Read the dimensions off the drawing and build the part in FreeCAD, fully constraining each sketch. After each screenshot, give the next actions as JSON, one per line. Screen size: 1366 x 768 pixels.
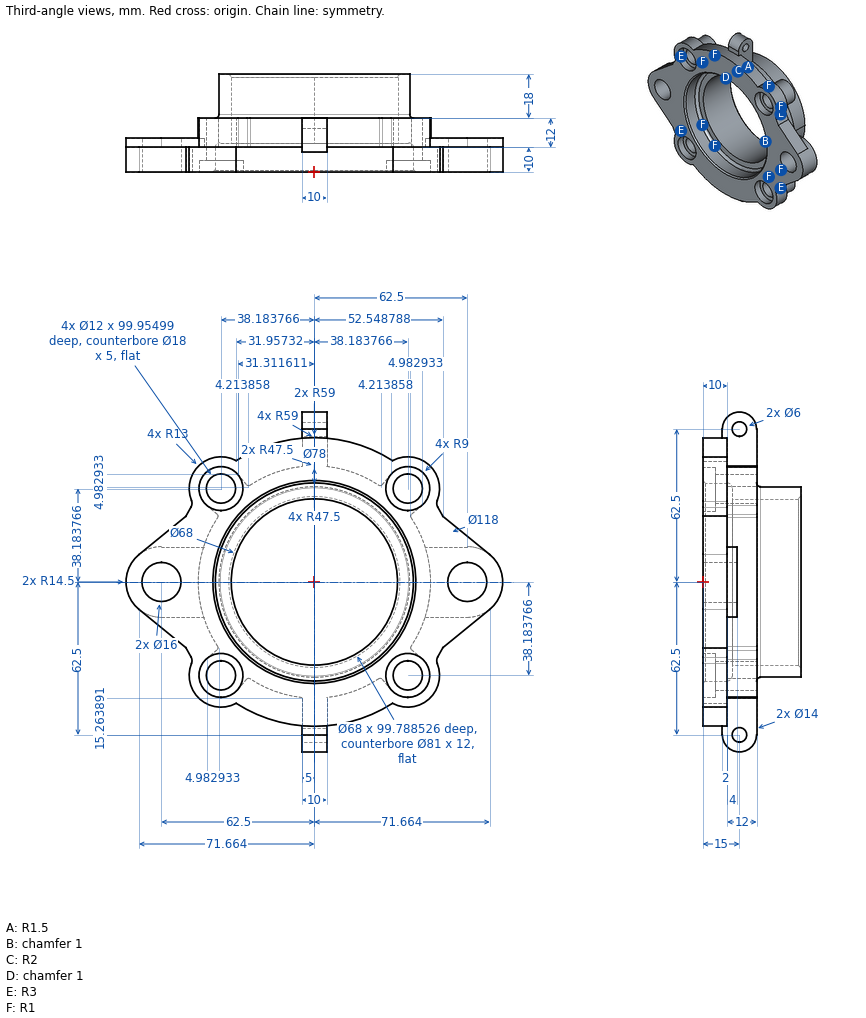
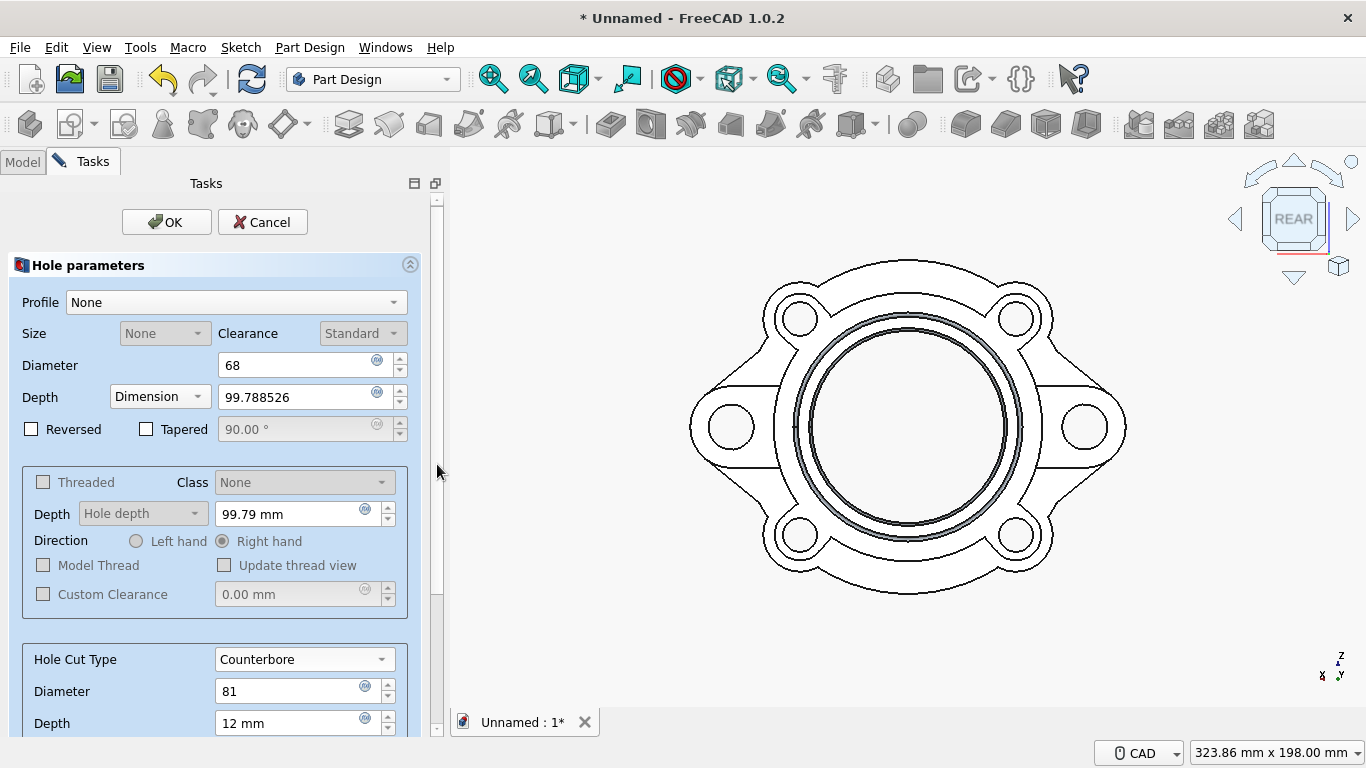
{"action": "left_click", "coordinate": [167, 222]}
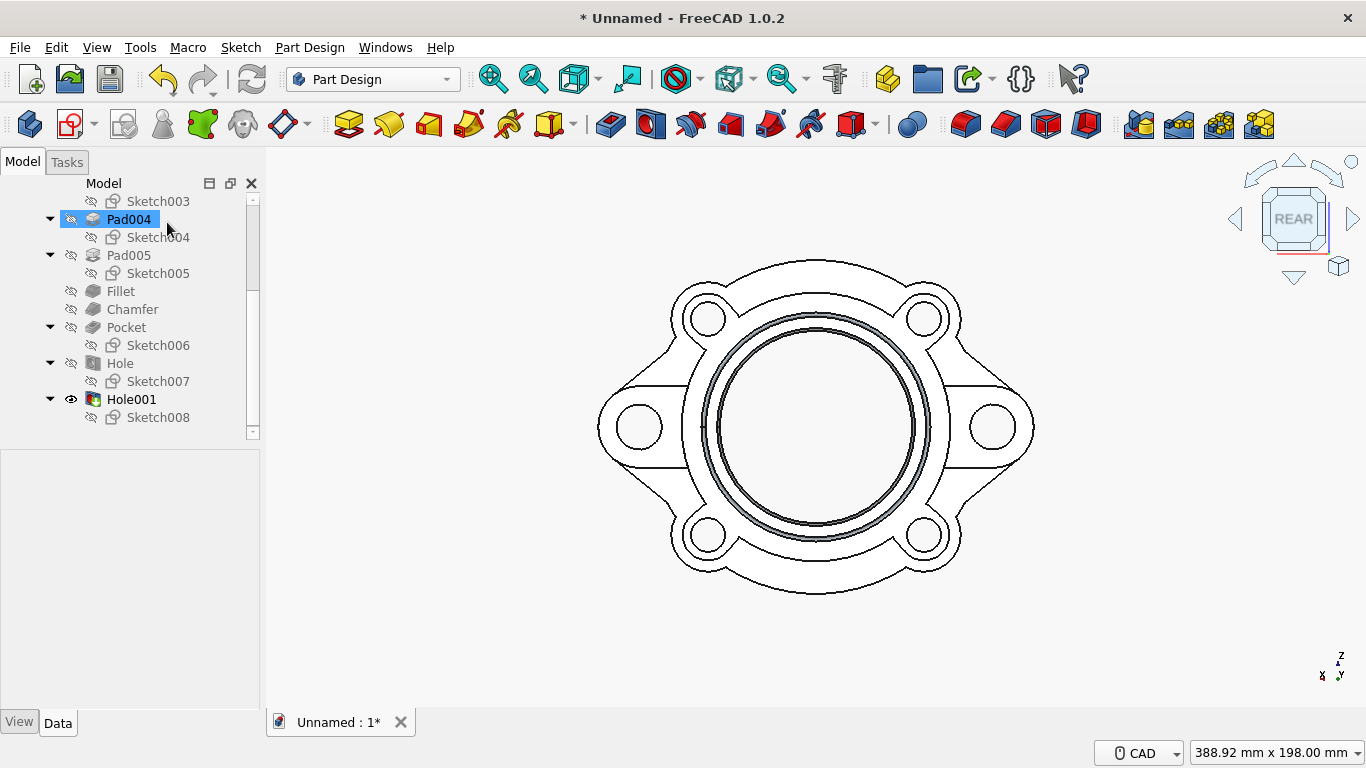
{"action": "key", "text": "0"}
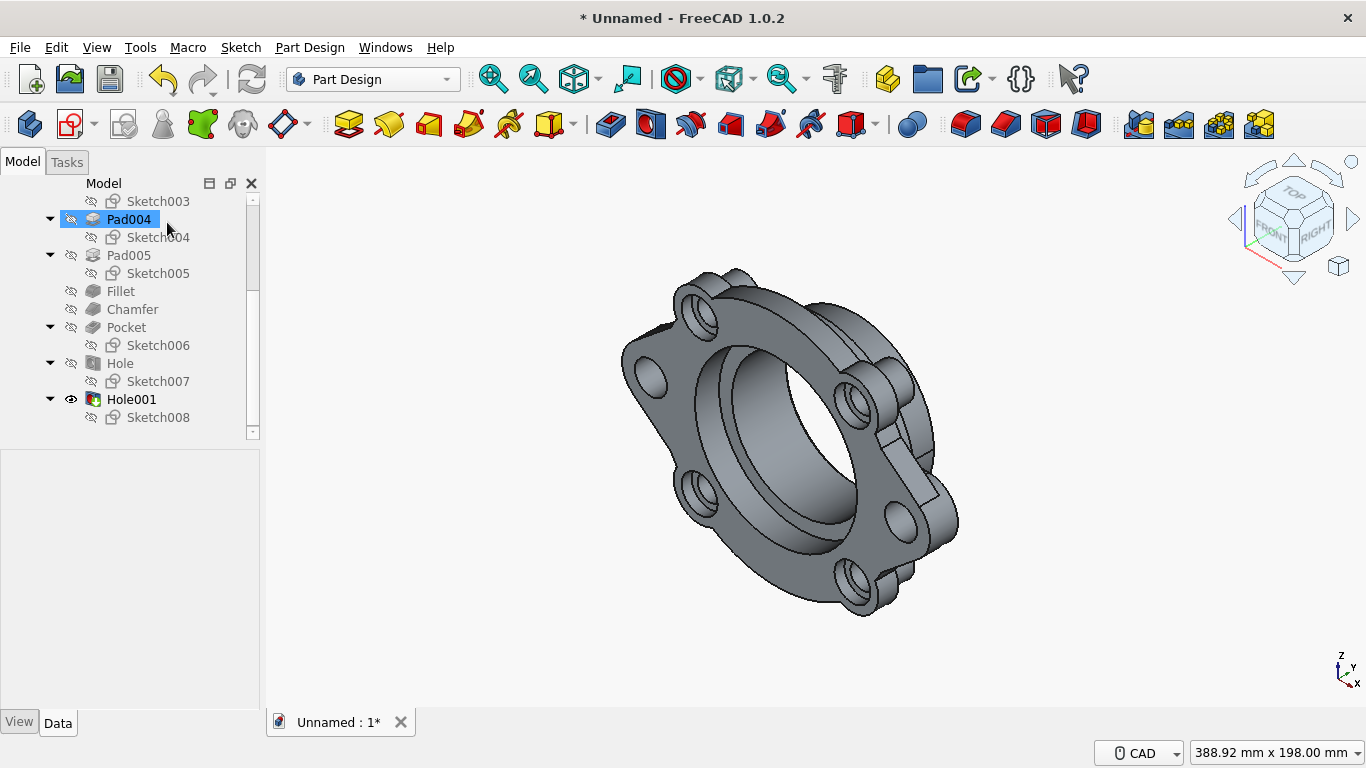
{"action": "key", "text": "2"}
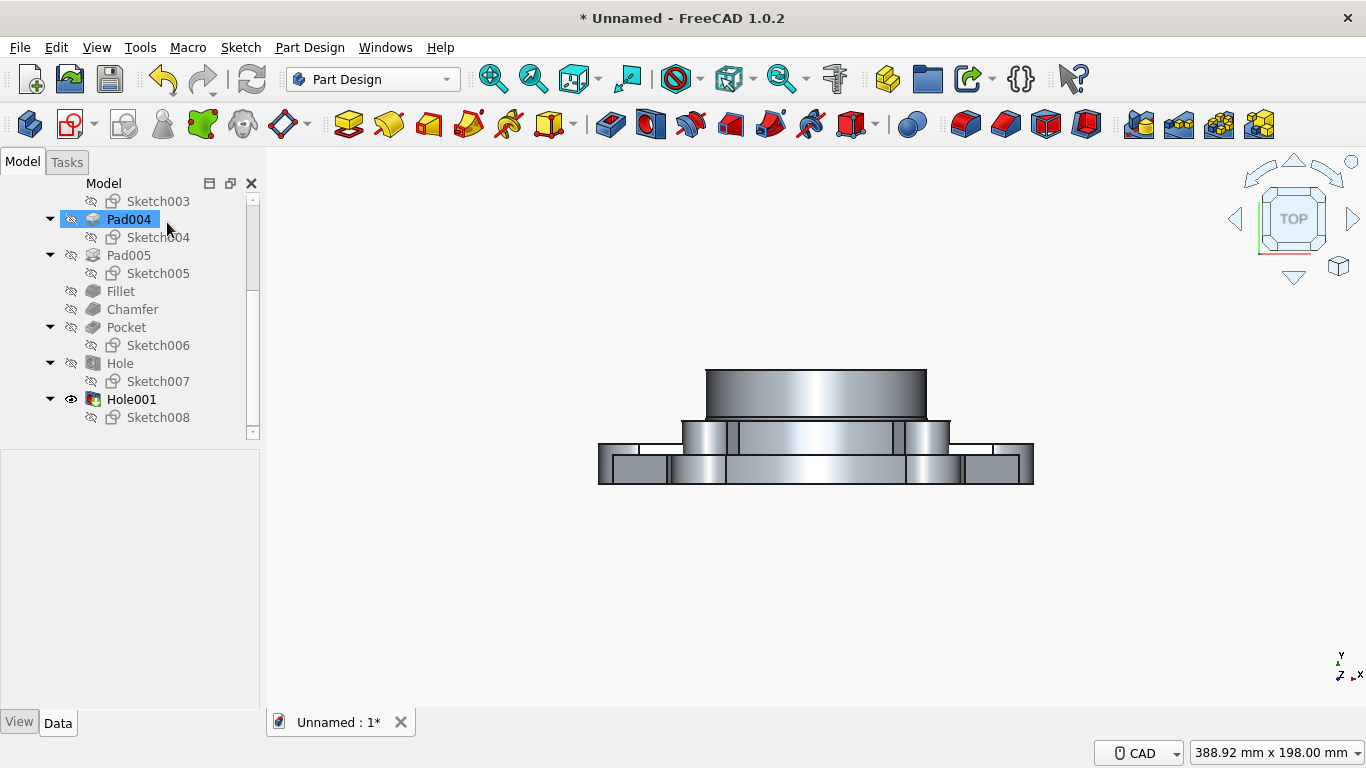
{"action": "left_click", "coordinate": [494, 80]}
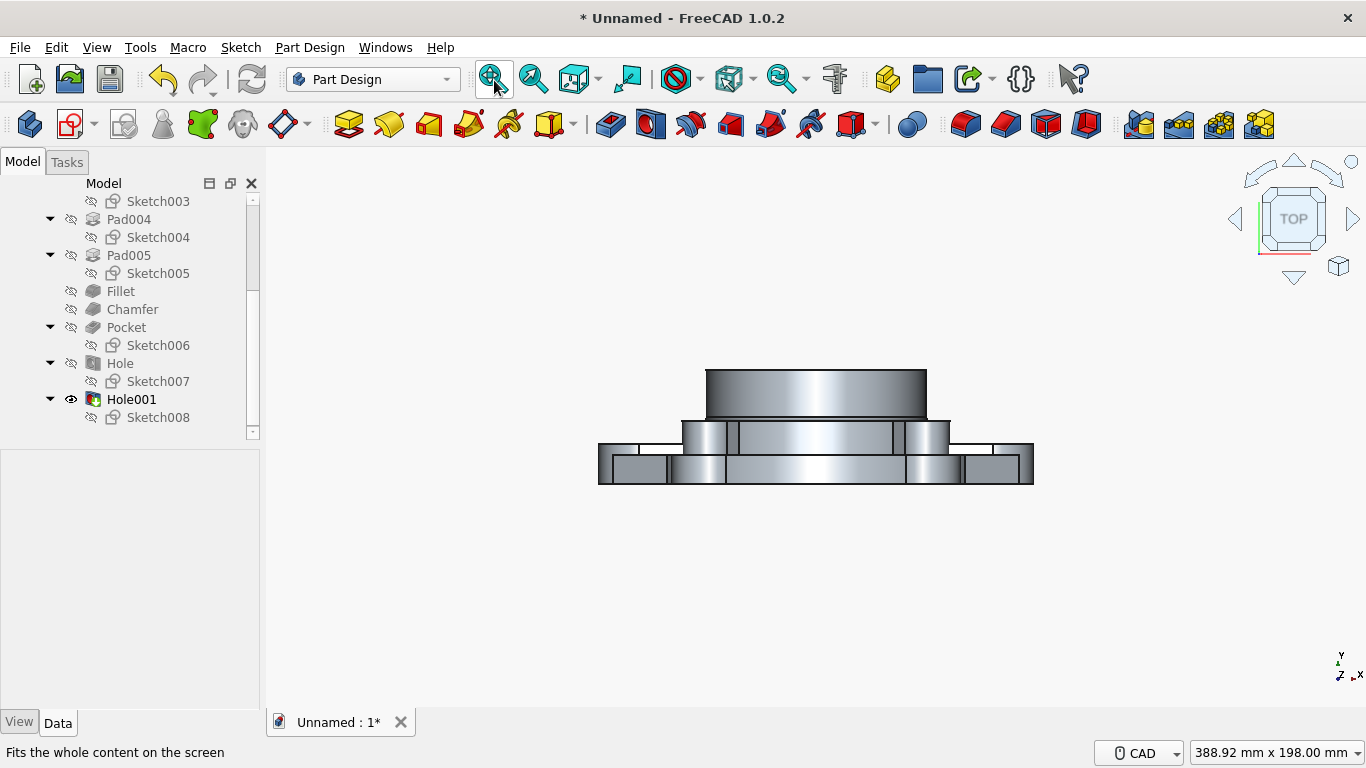
{"action": "key", "text": "1"}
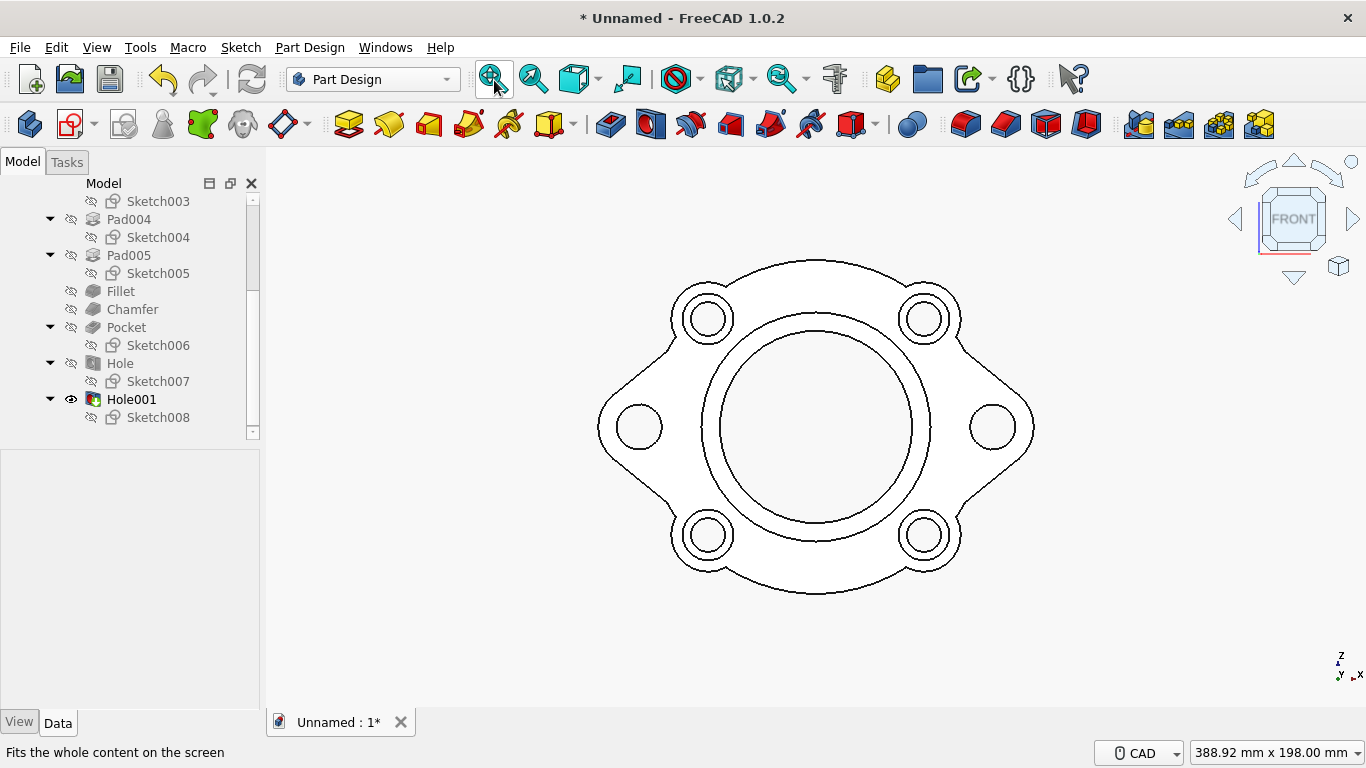
{"action": "key", "text": "3"}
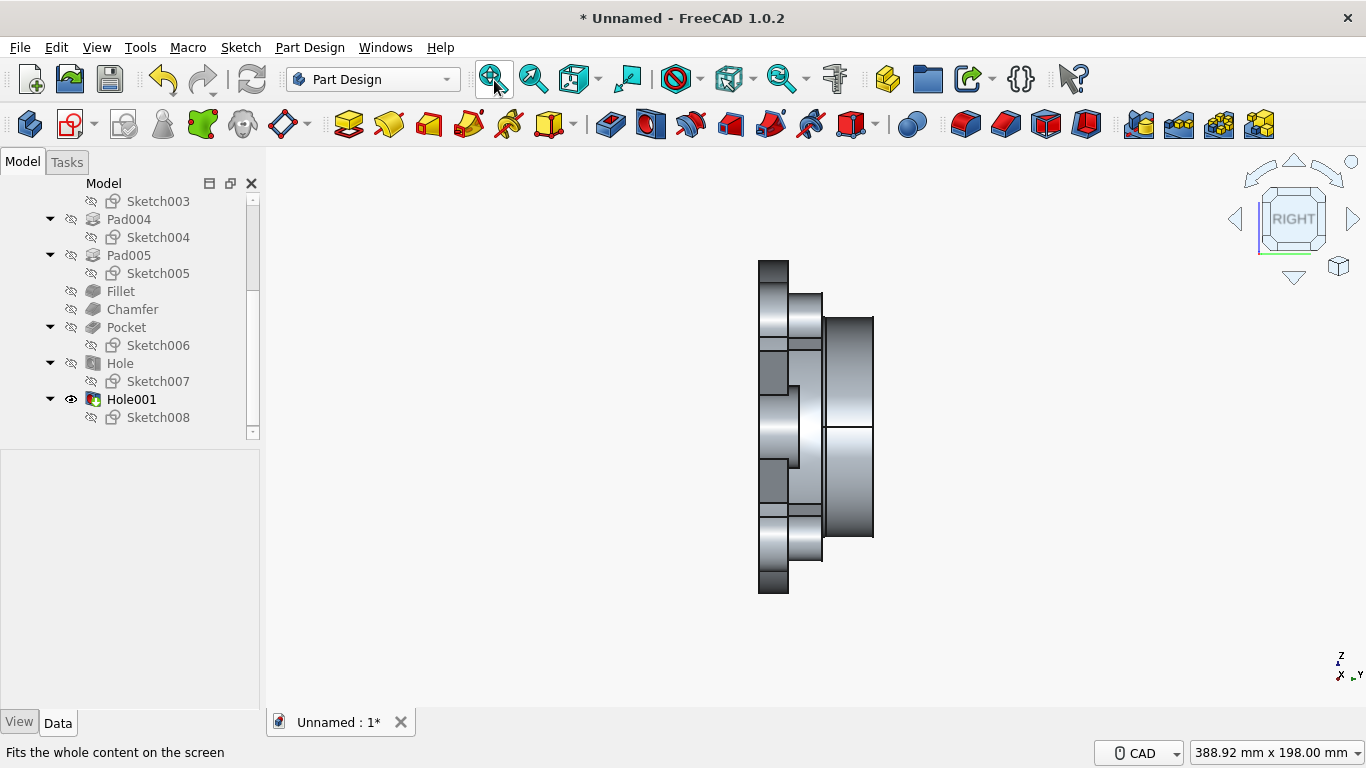
{"action": "key", "text": "5"}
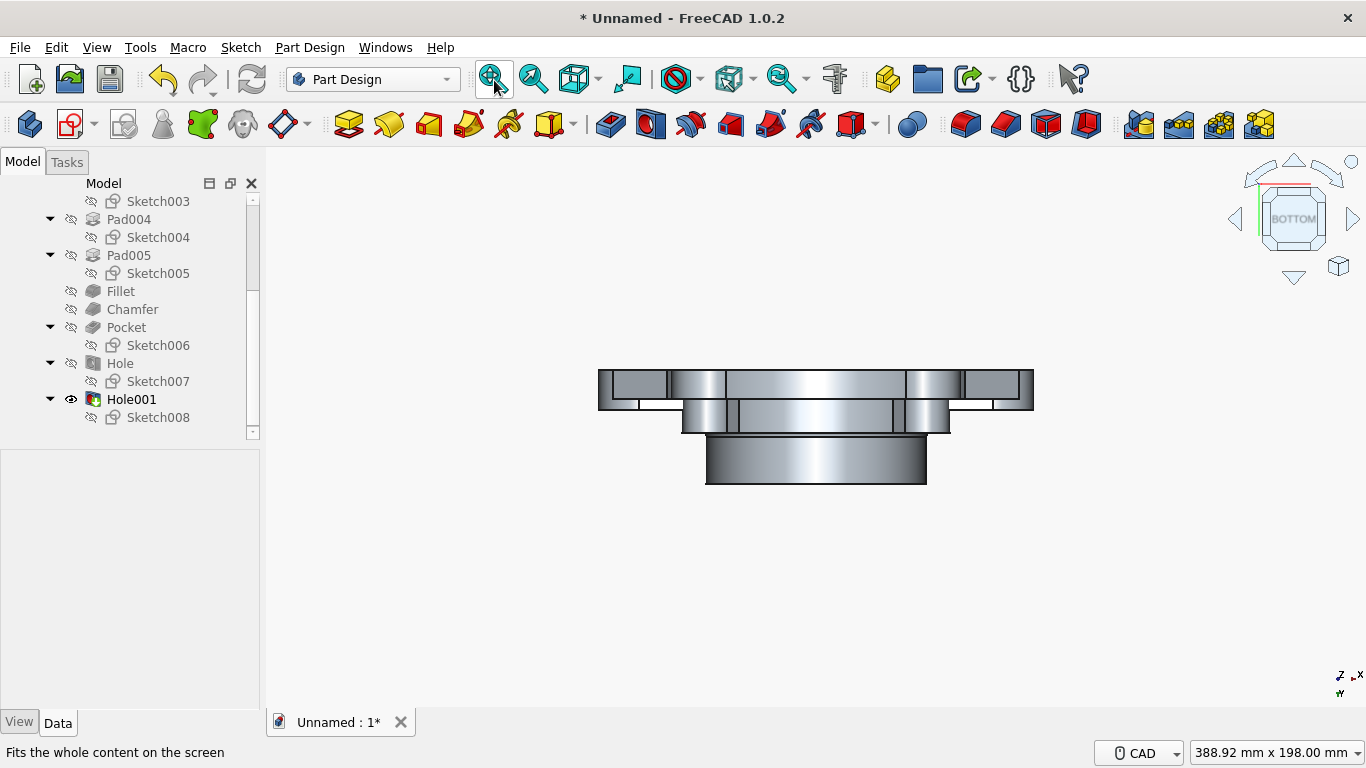
{"action": "left_click", "coordinate": [494, 80]}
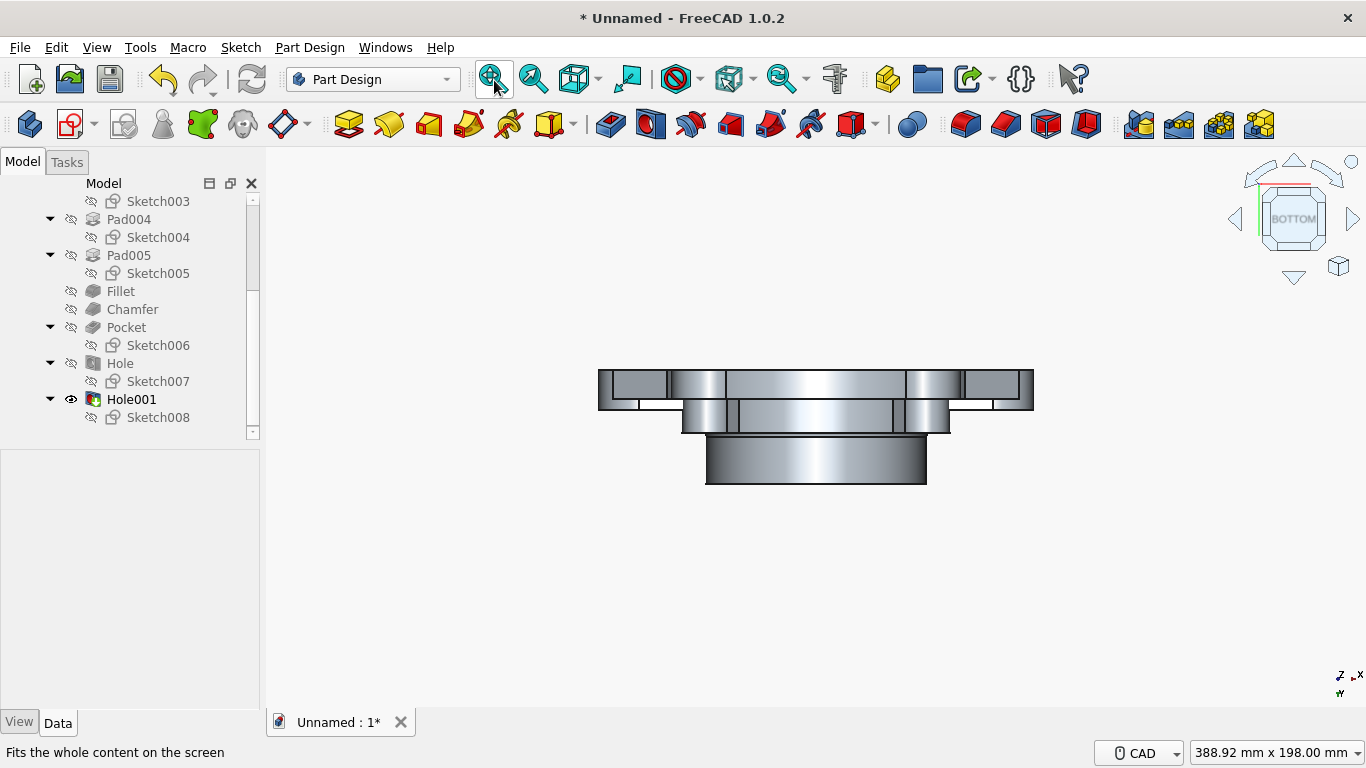
{"action": "key", "text": "4"}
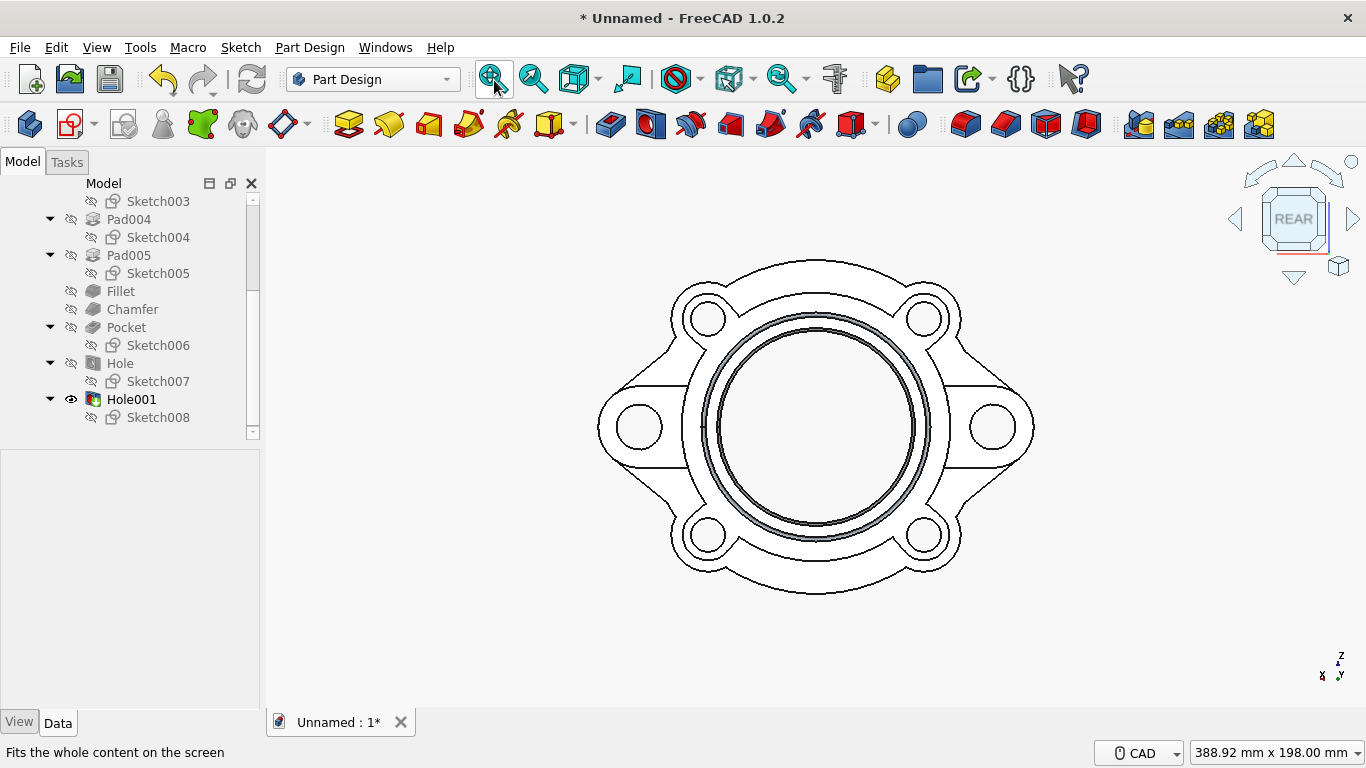
{"action": "key", "text": "6"}